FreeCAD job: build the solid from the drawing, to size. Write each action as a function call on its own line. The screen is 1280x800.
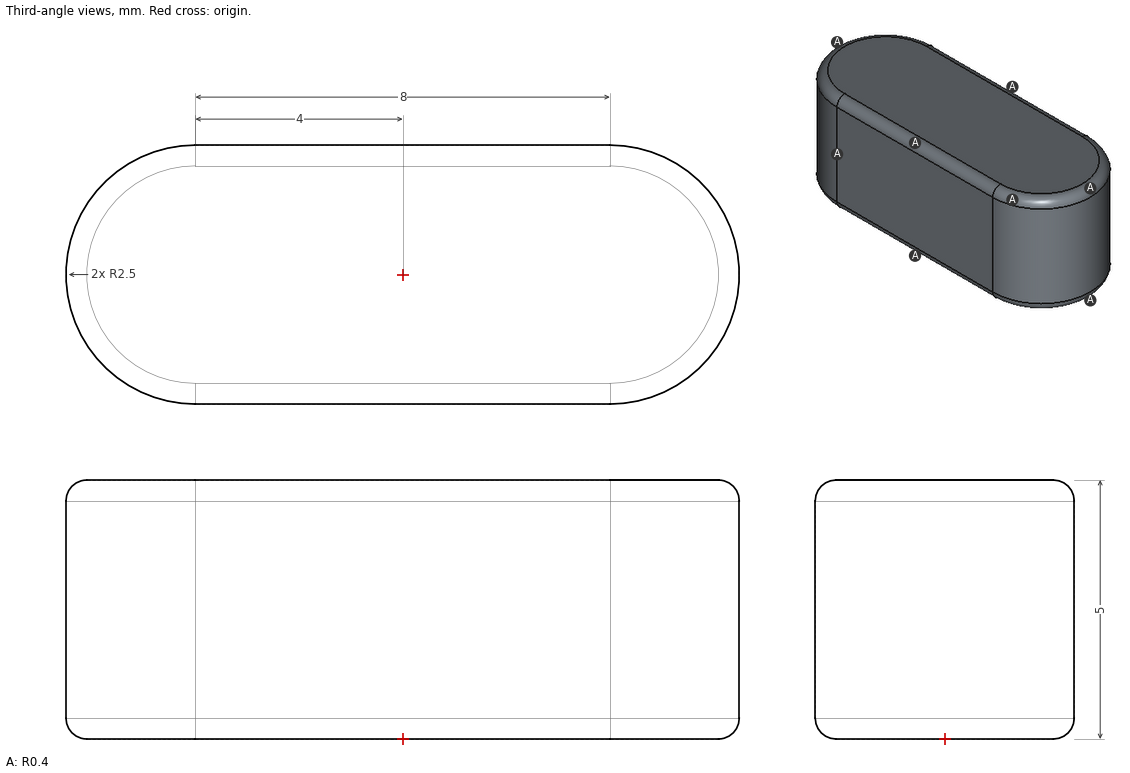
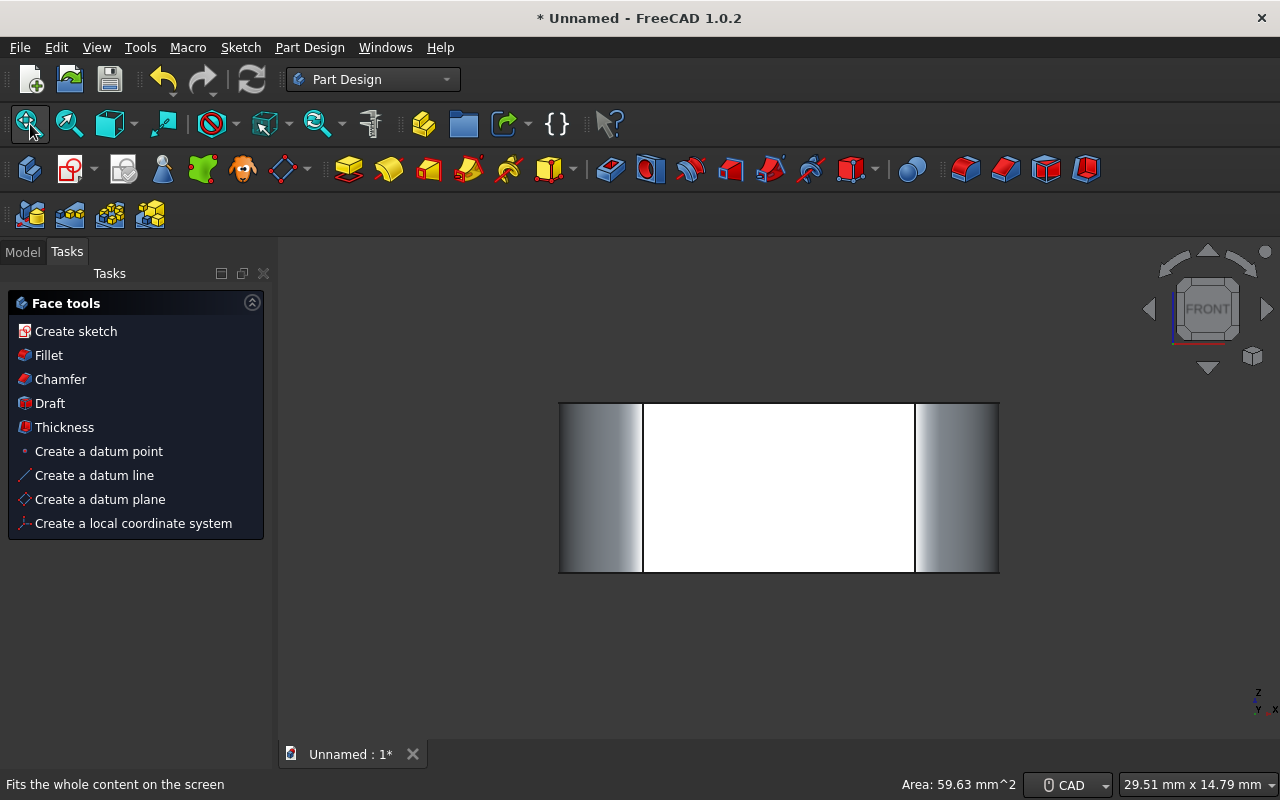
key(3)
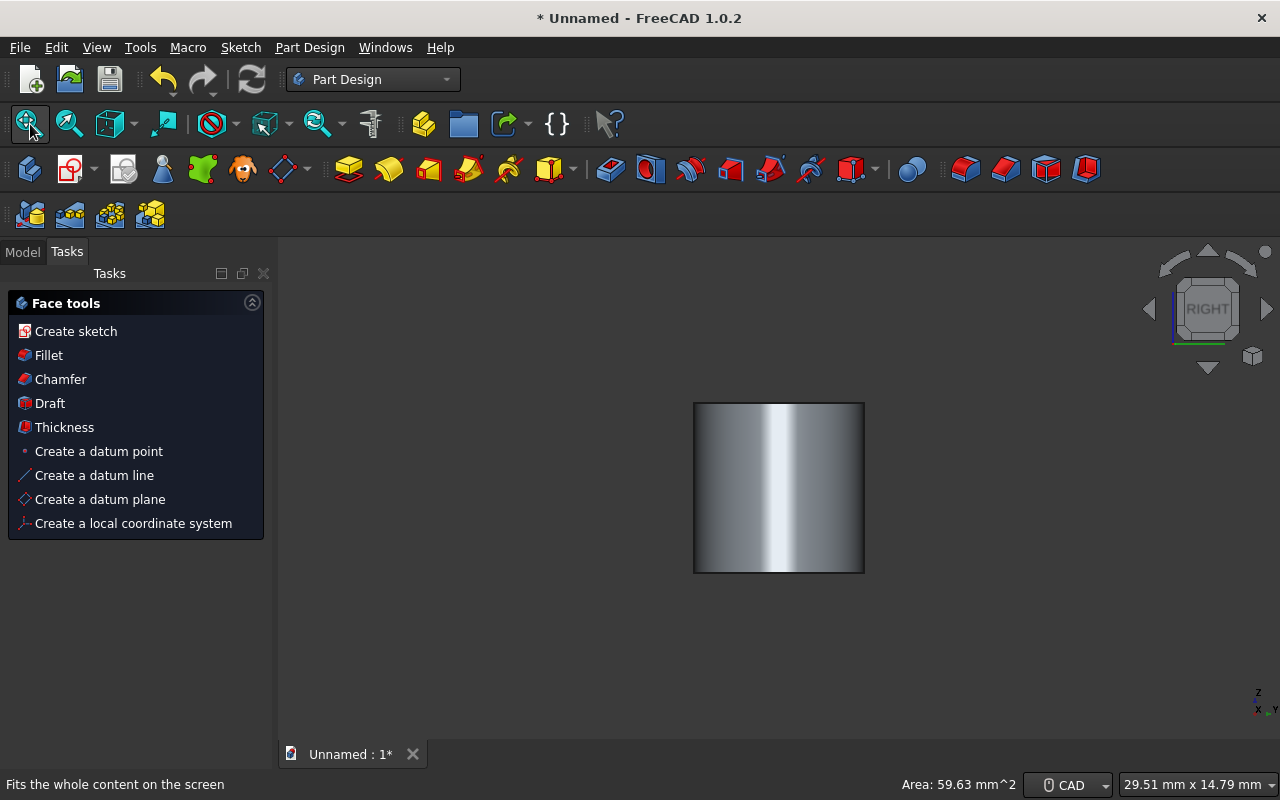
click(30, 124)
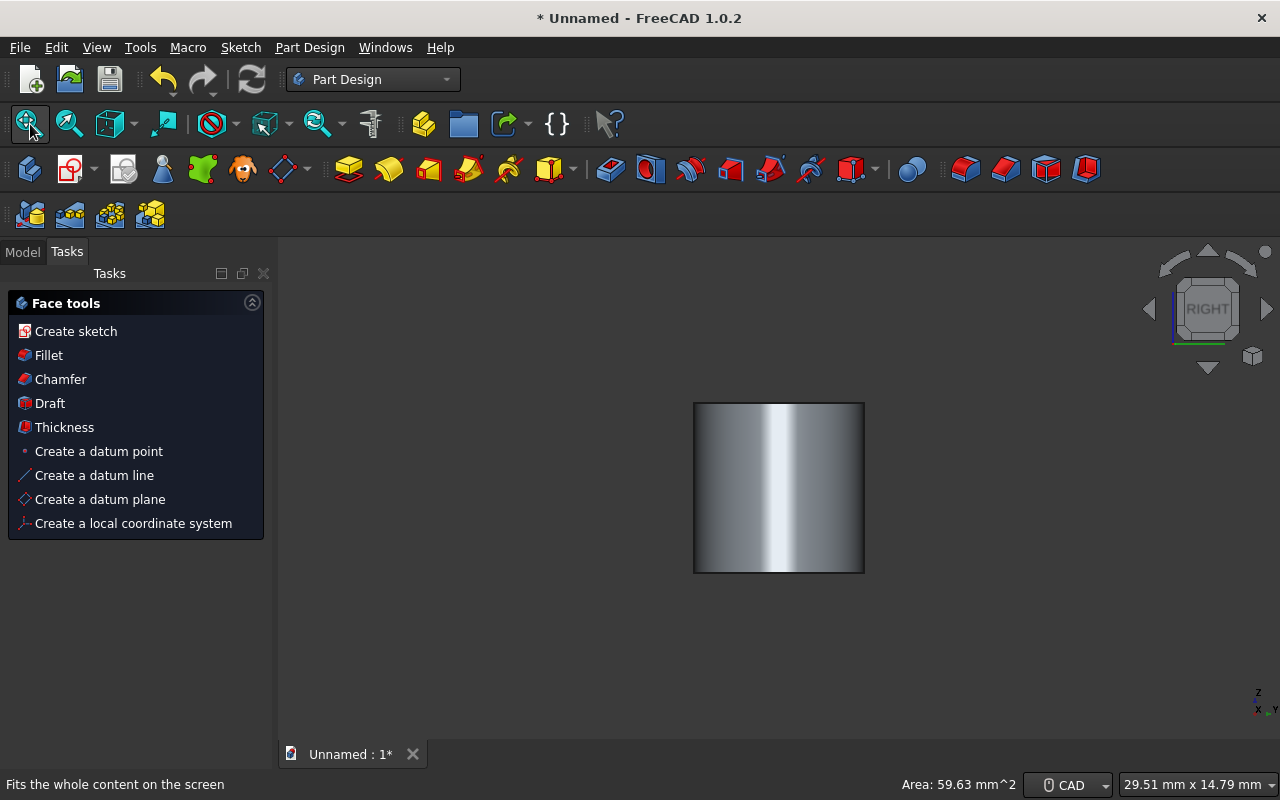
key(5)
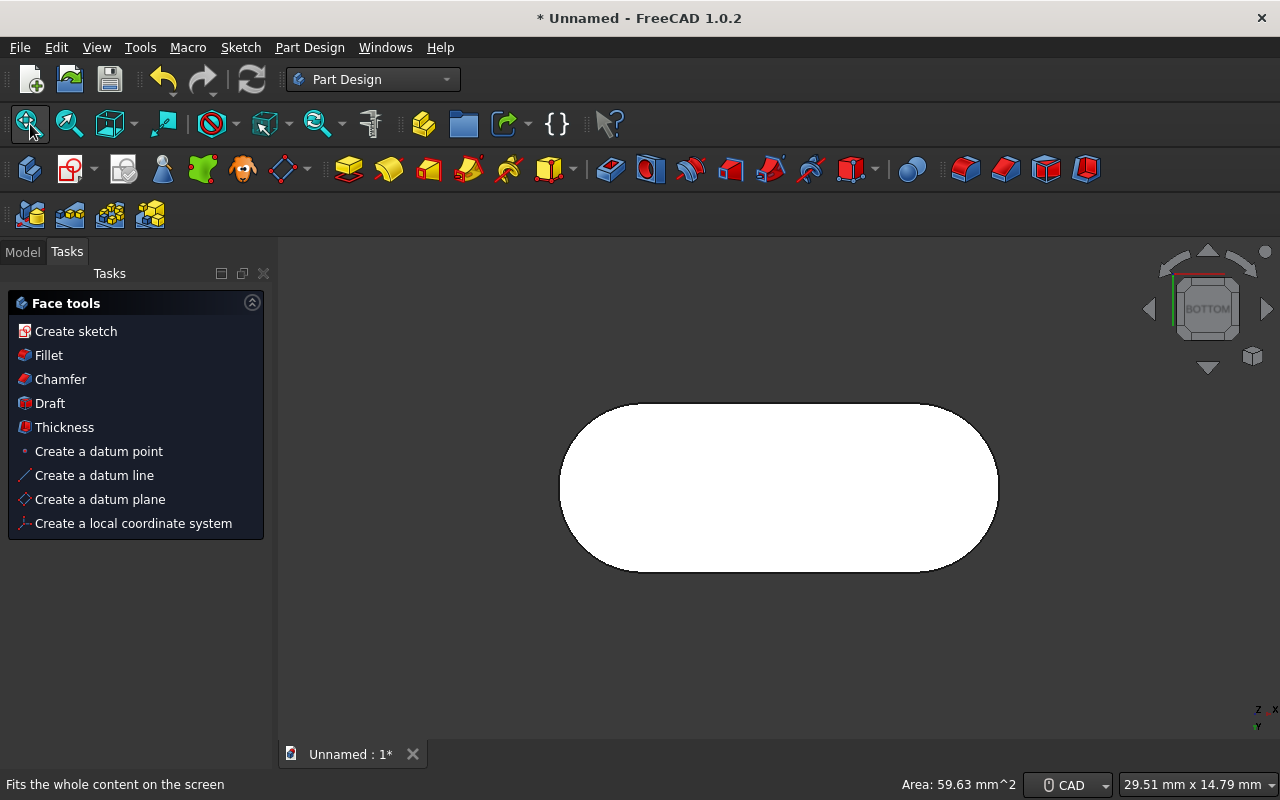
click(30, 124)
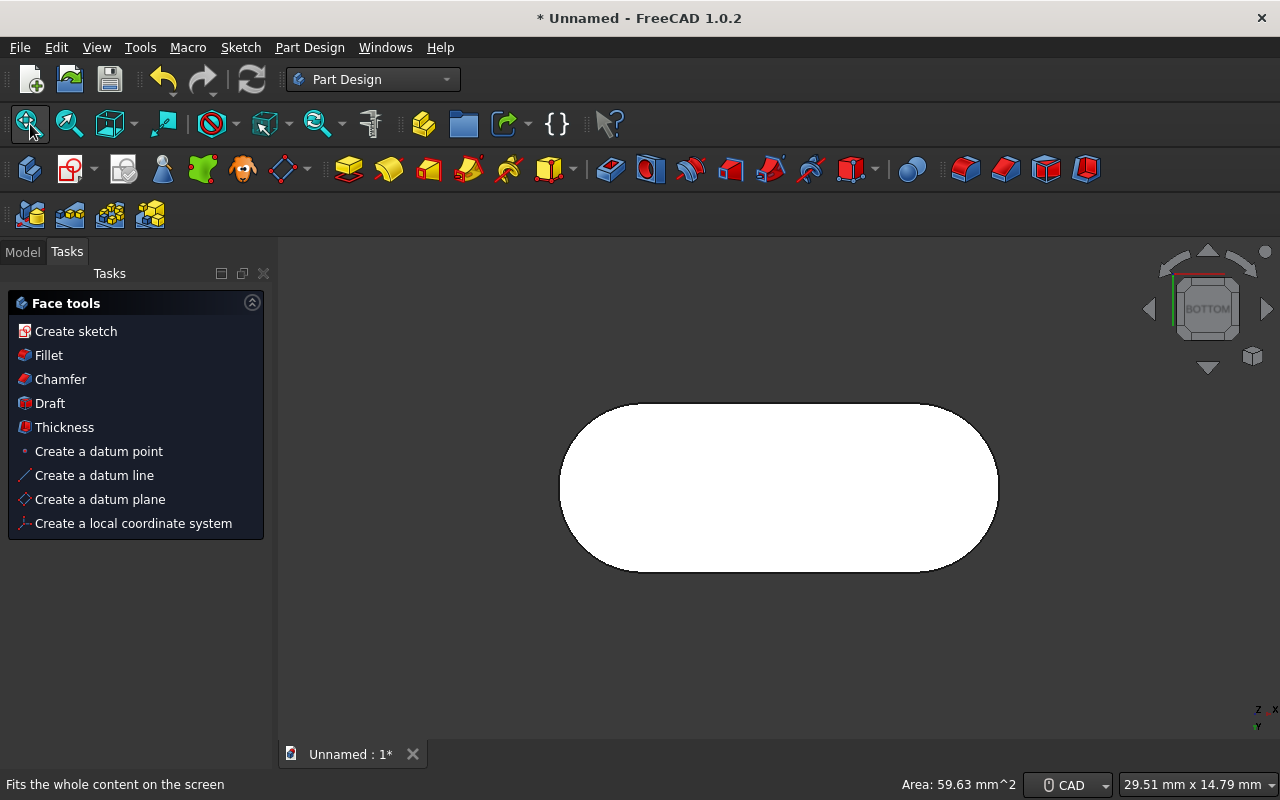
click(905, 487, ctrl)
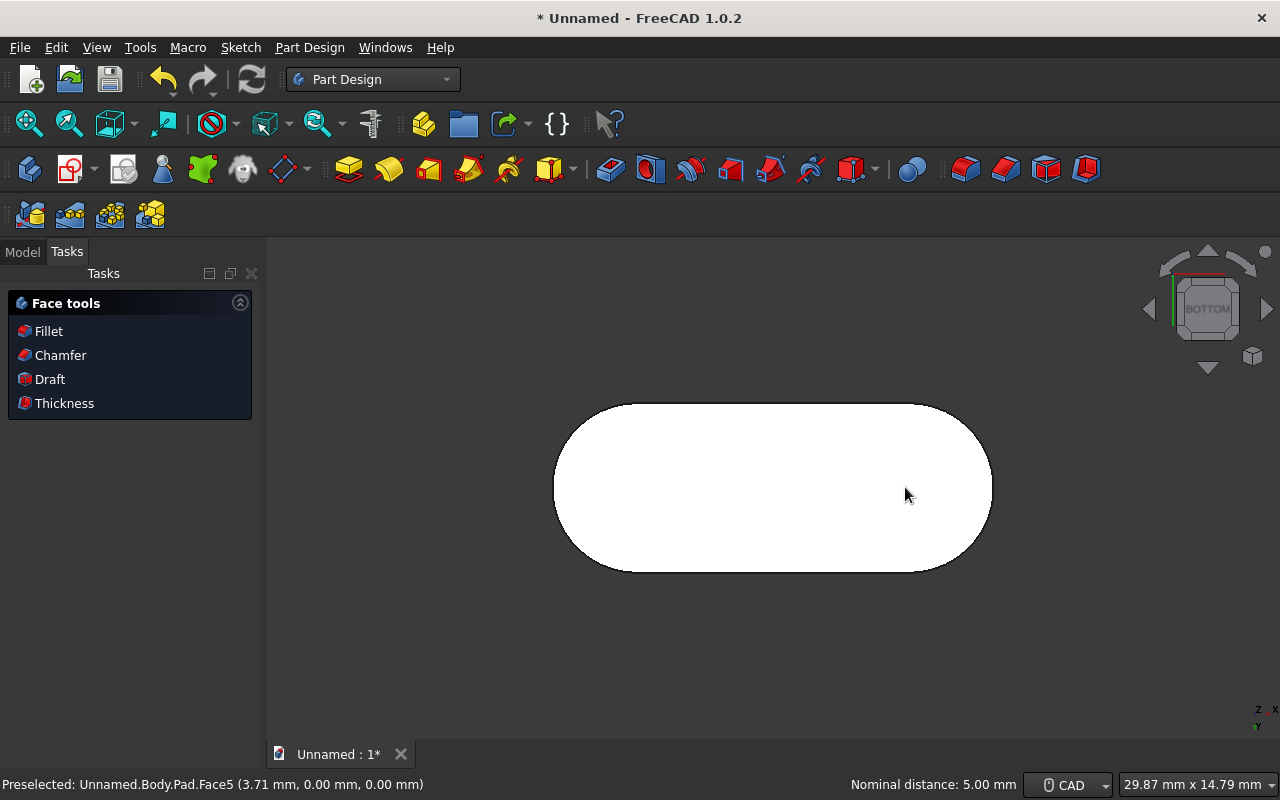
click(966, 170)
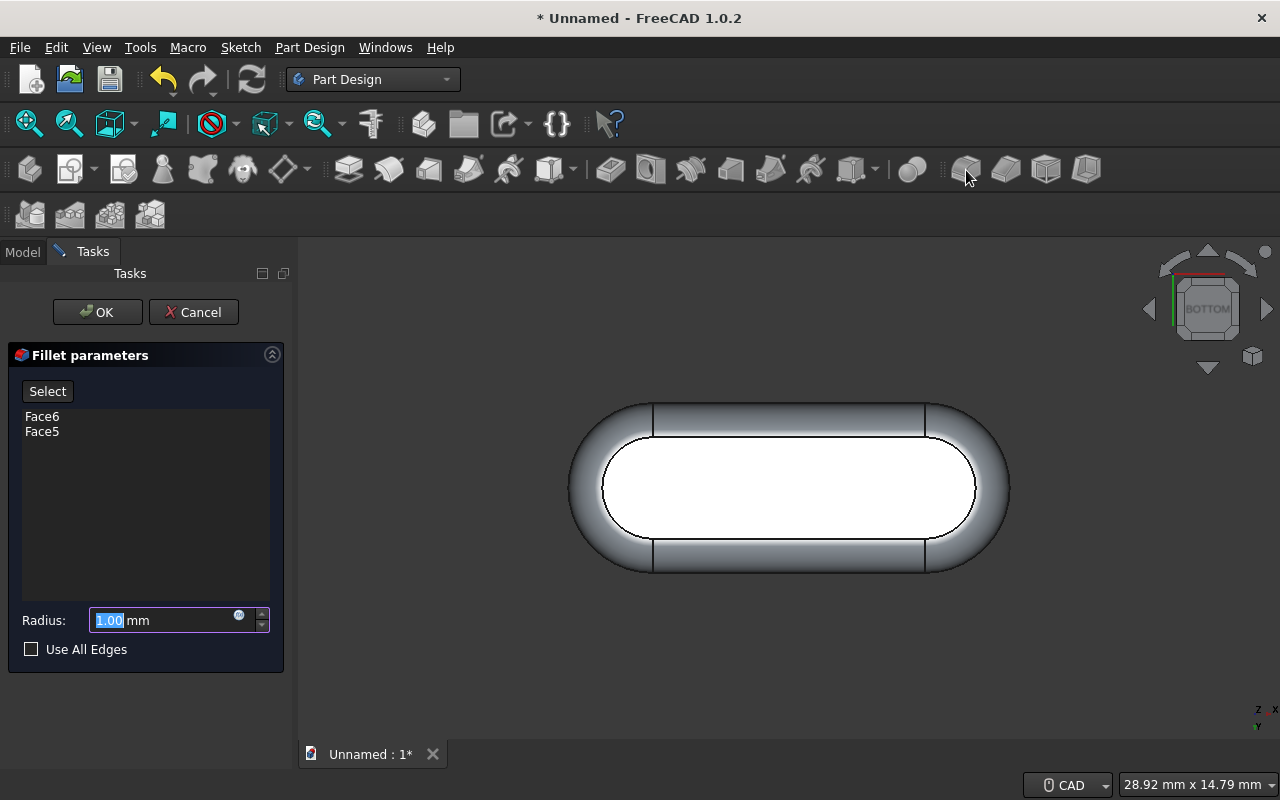
text(0.4)
key(Tab)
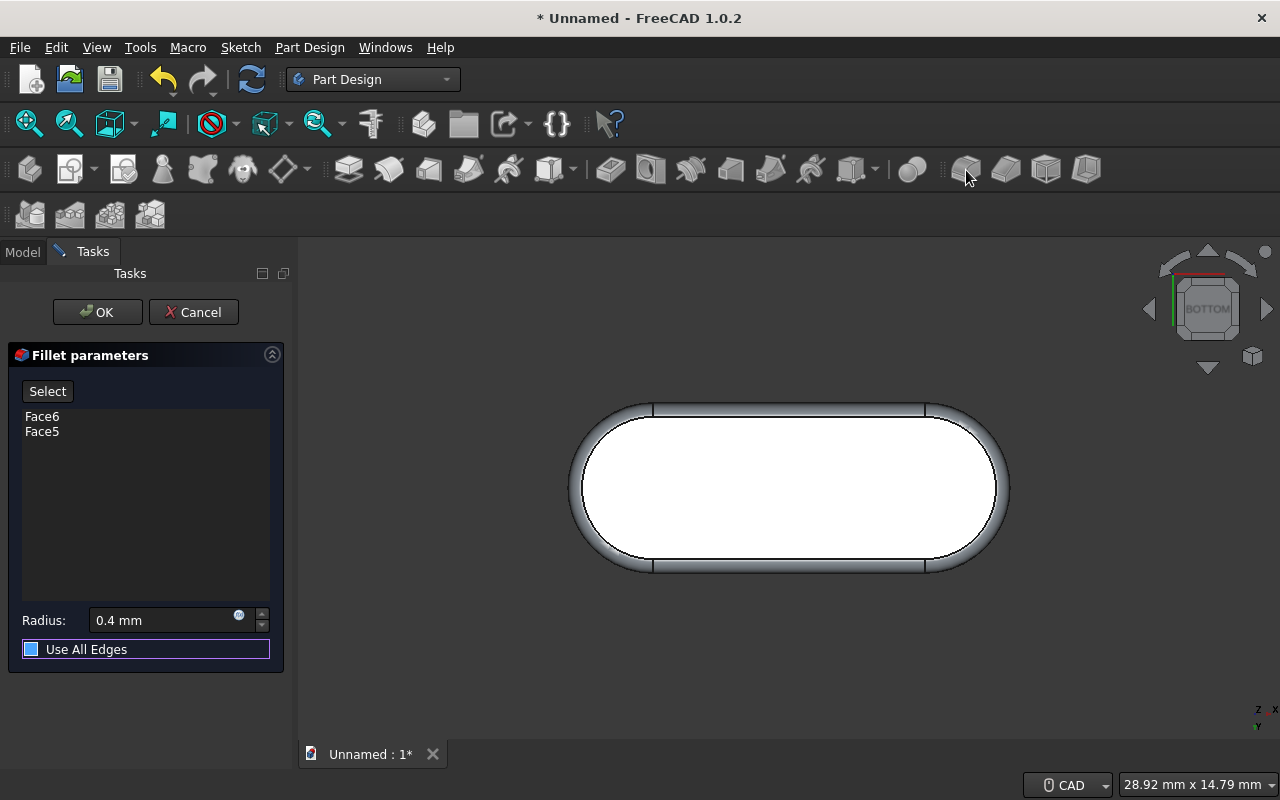
click(98, 312)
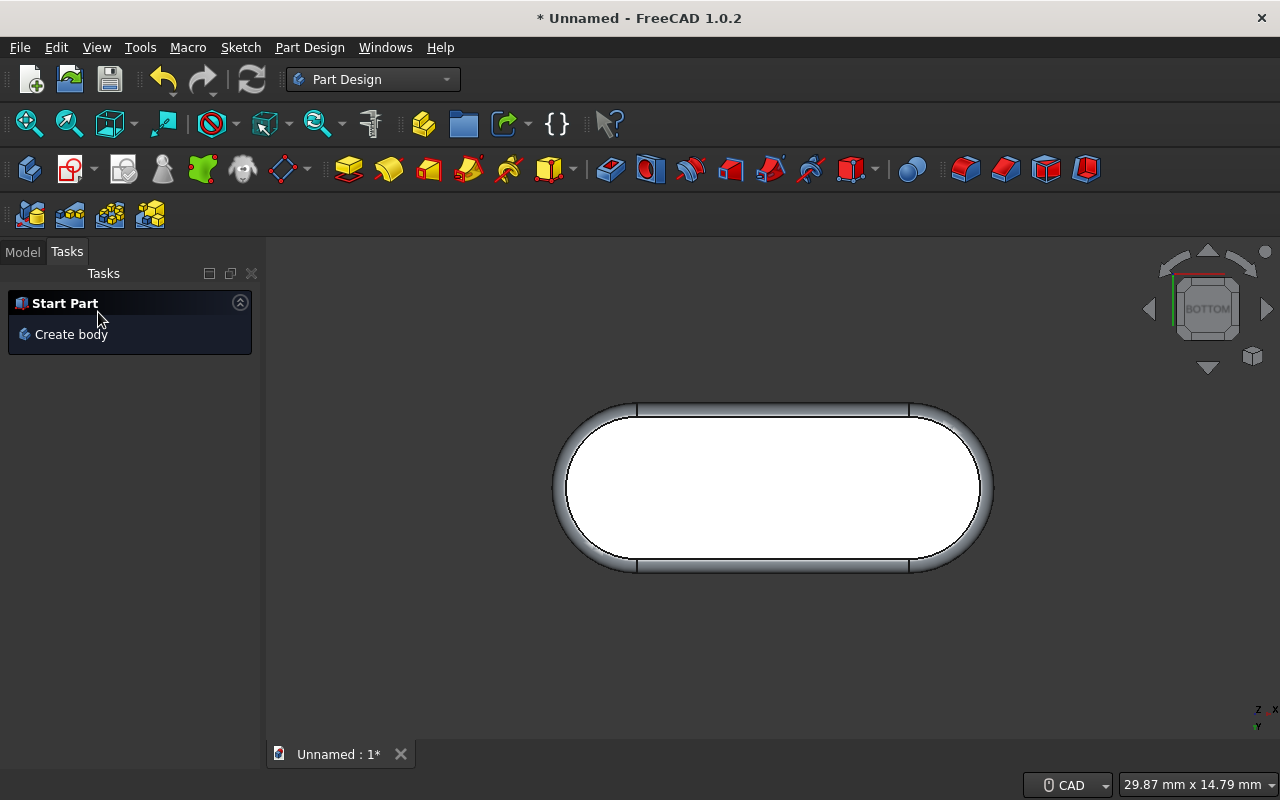
key(0)